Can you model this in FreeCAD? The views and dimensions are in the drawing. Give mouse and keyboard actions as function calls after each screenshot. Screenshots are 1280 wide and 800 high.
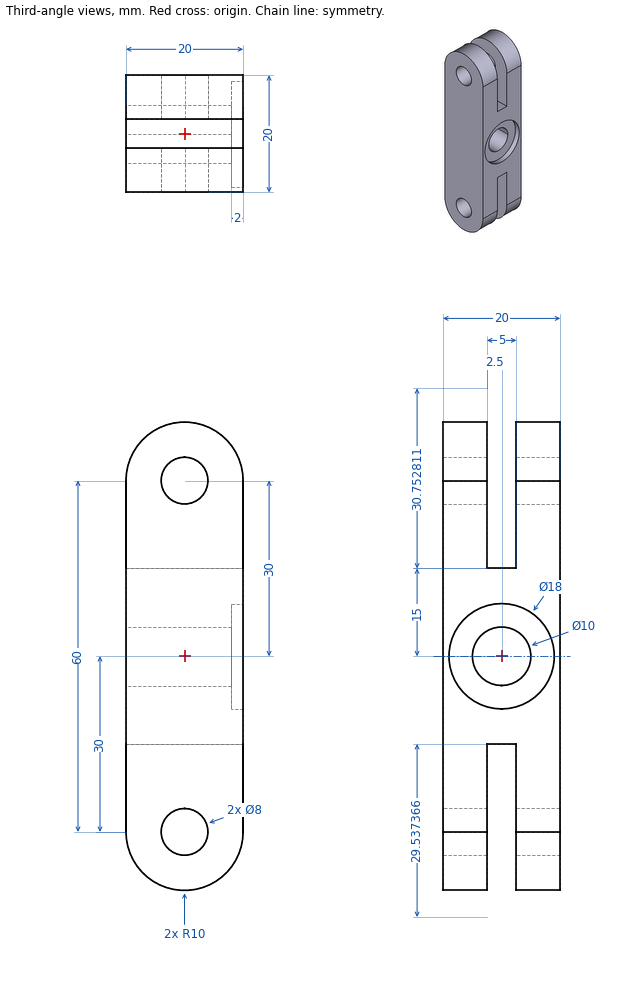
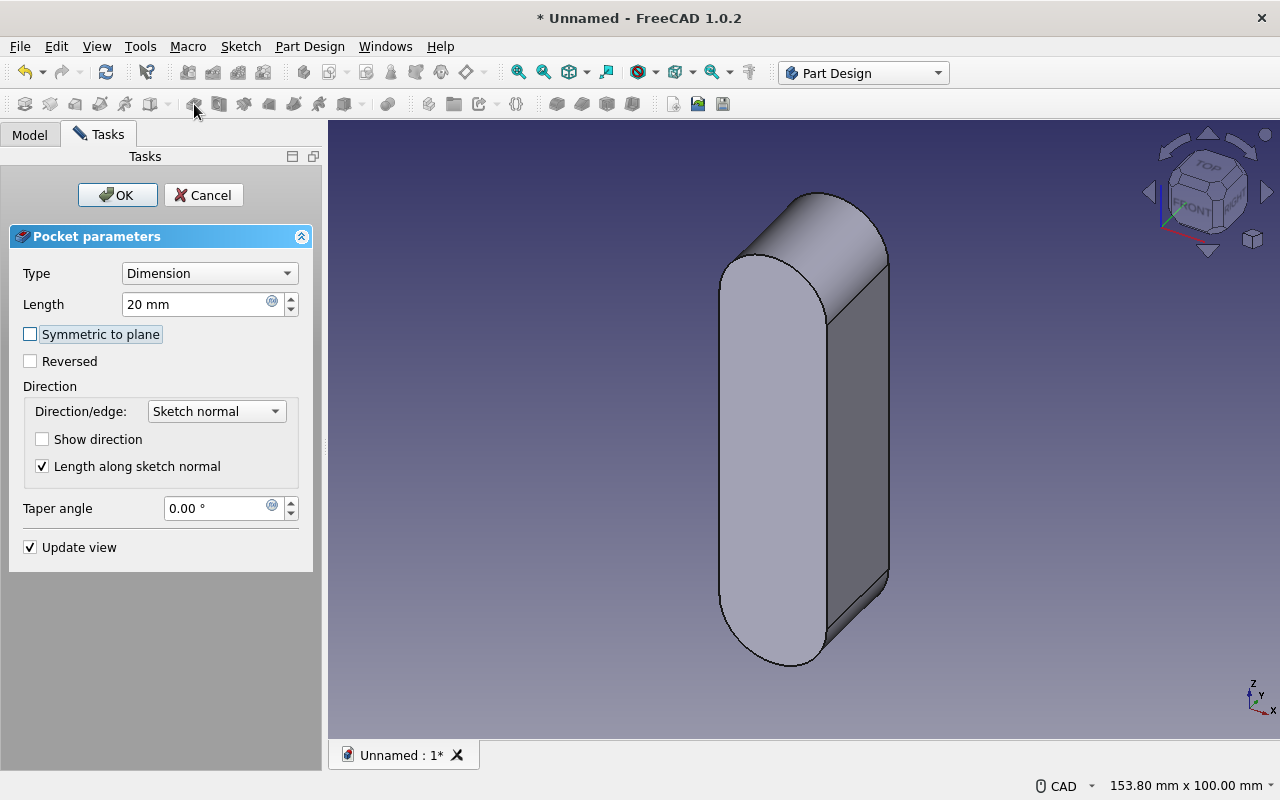
click(31, 334)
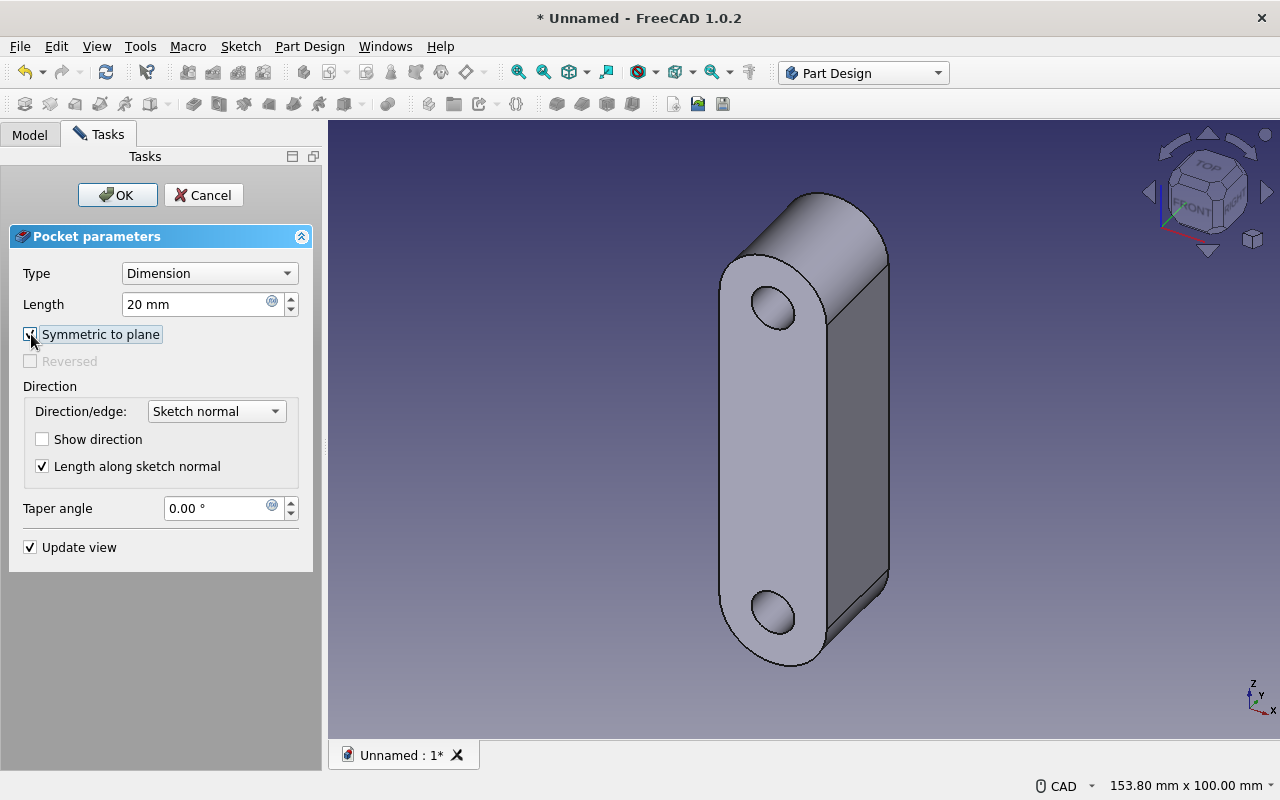
click(118, 195)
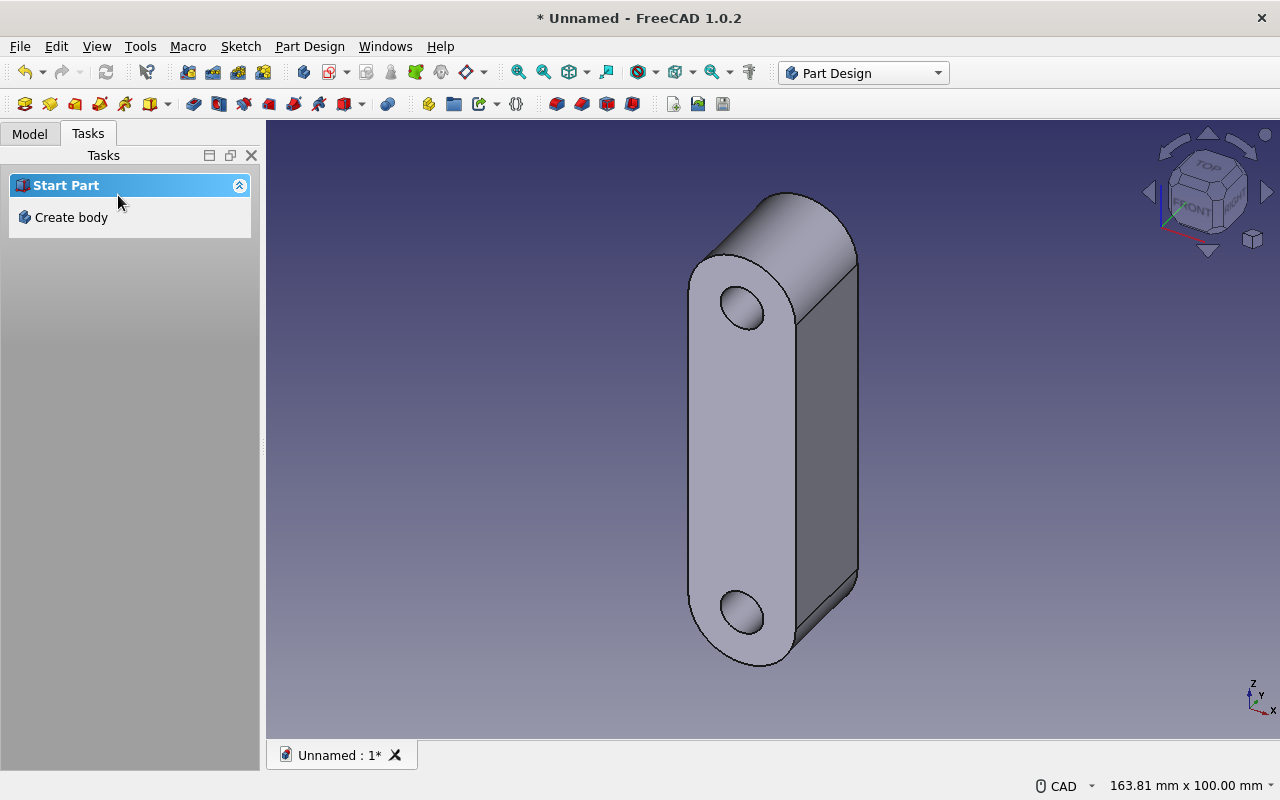
click(328, 72)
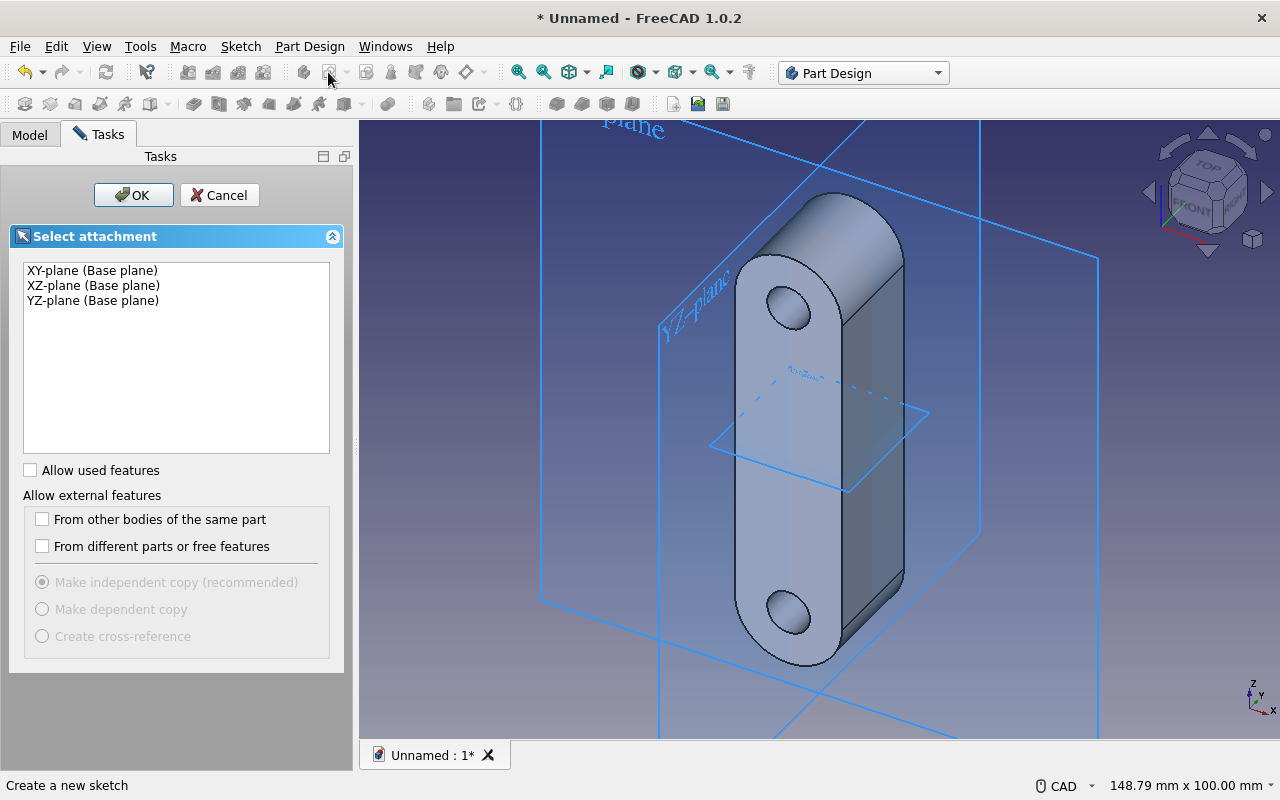
click(84, 300)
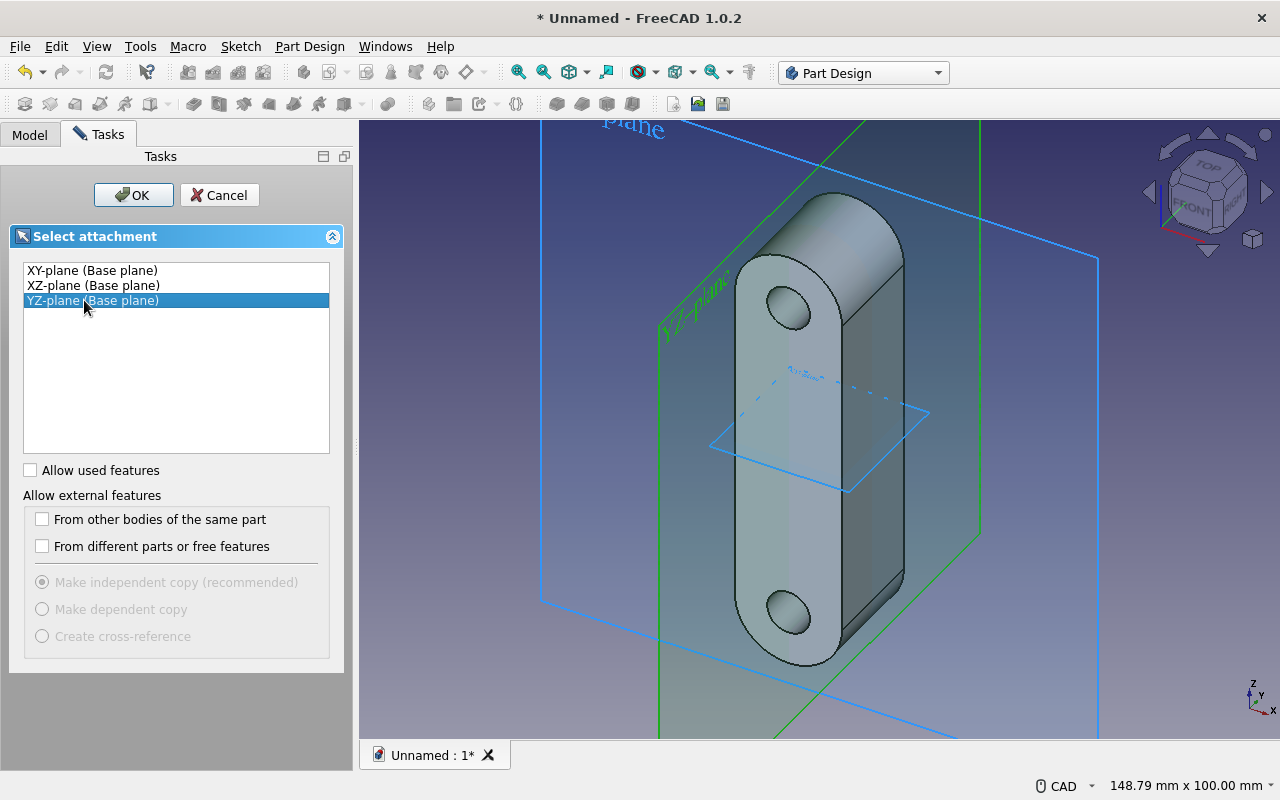
click(134, 195)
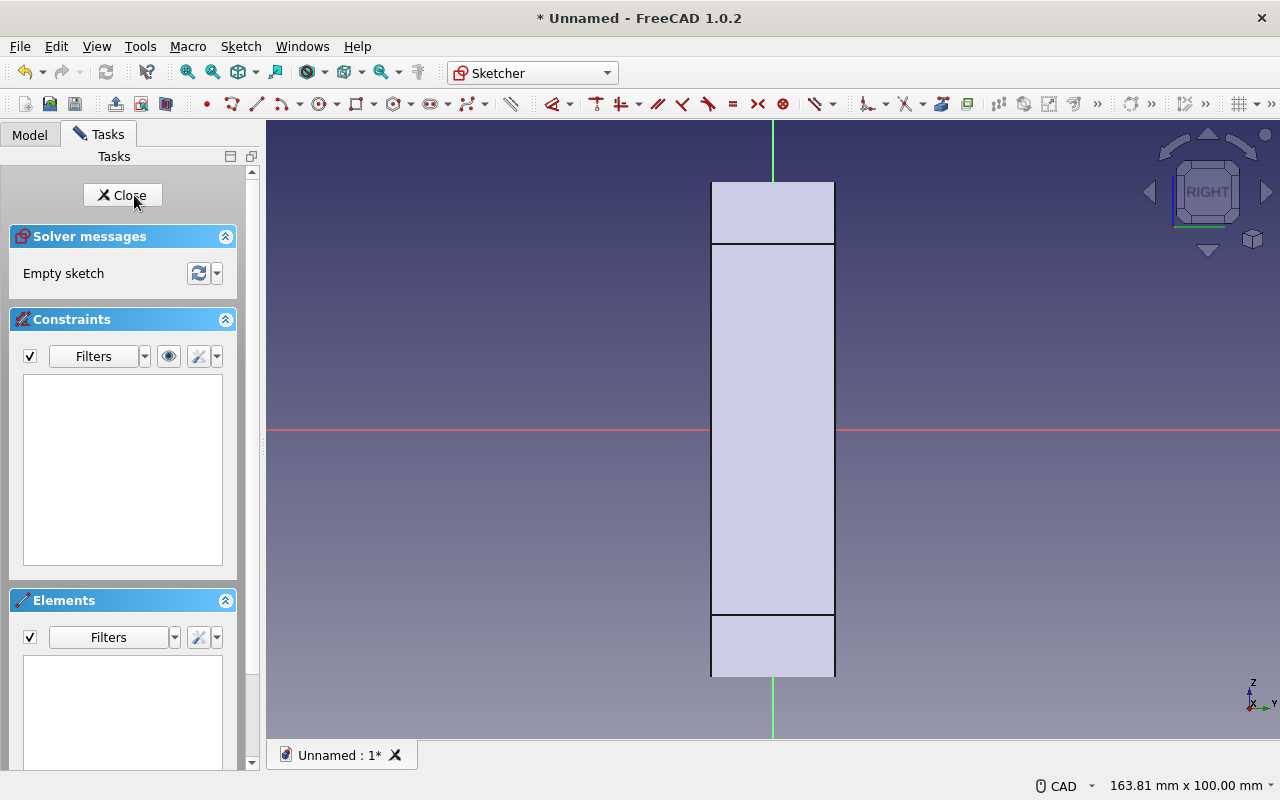
key(q)
key(s)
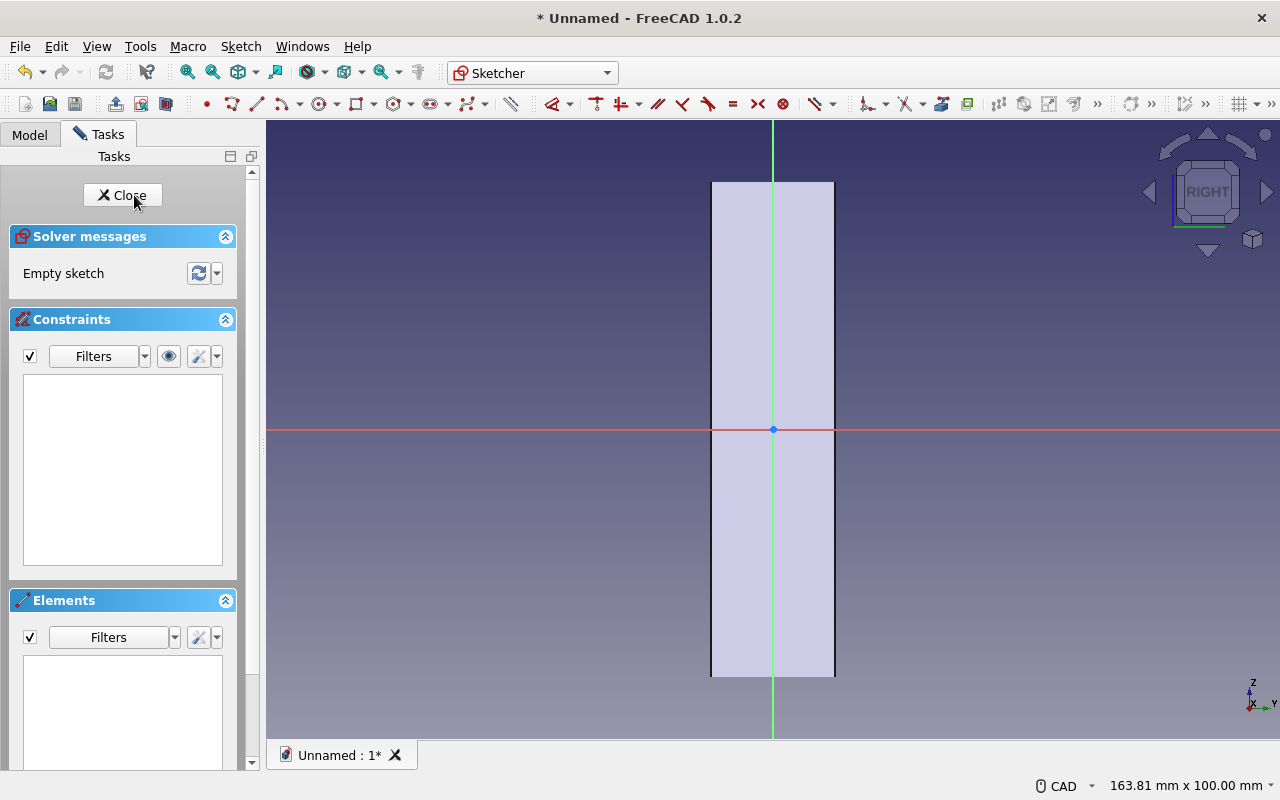
scroll(565, 437, down, 2)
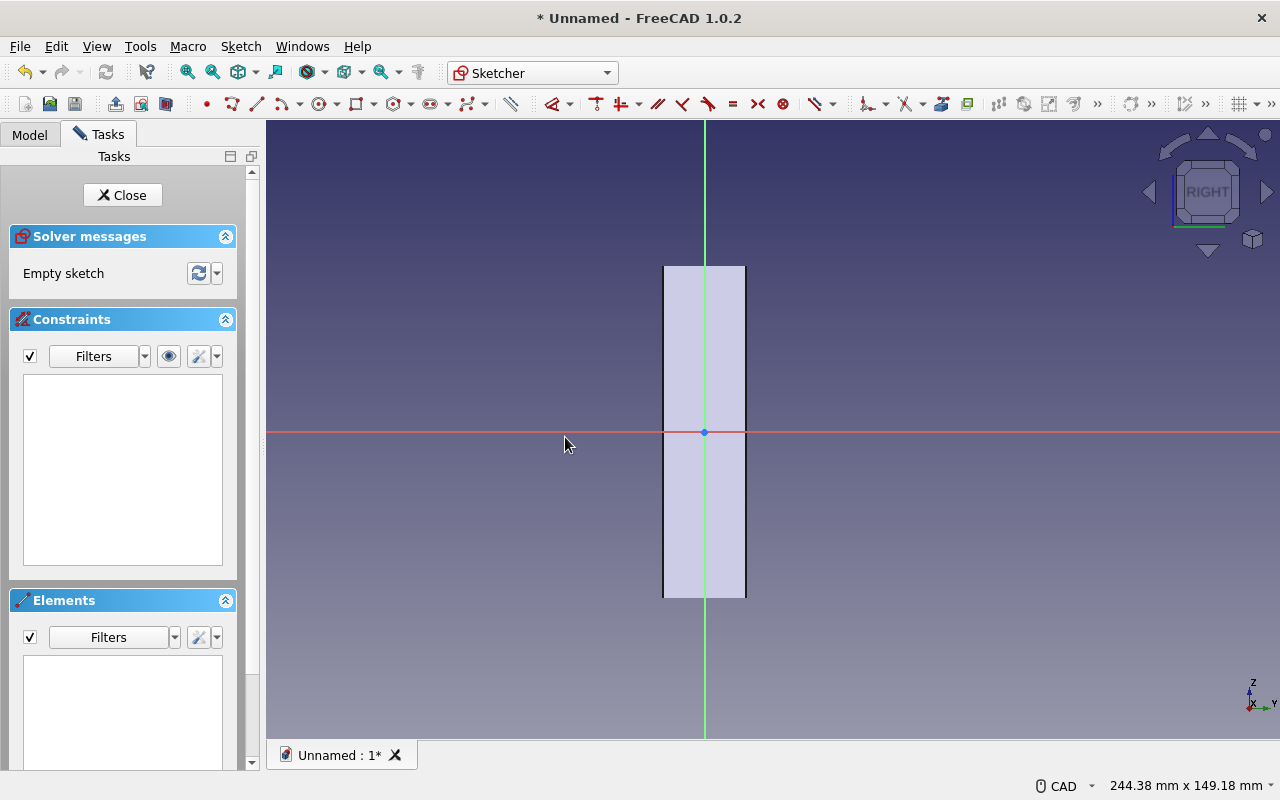
key(g)
key(r)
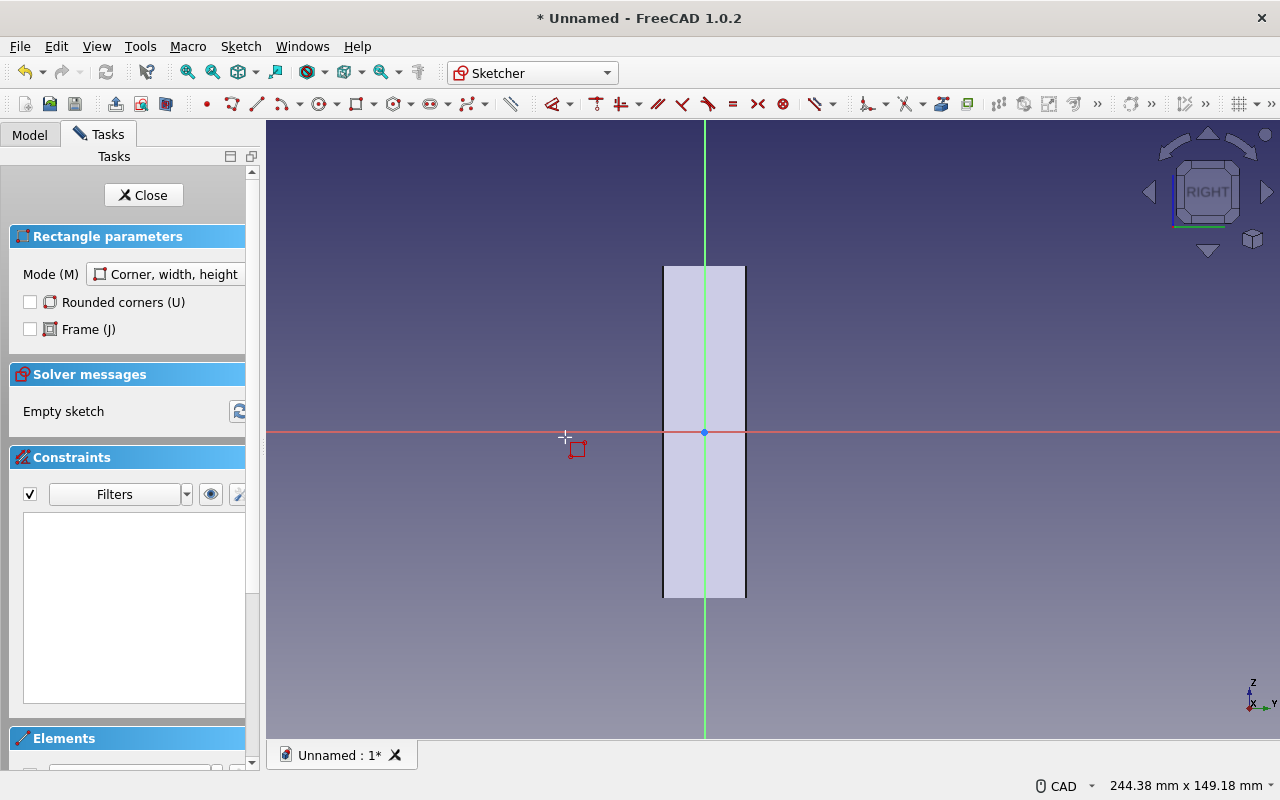
scroll(694, 242, up, 3)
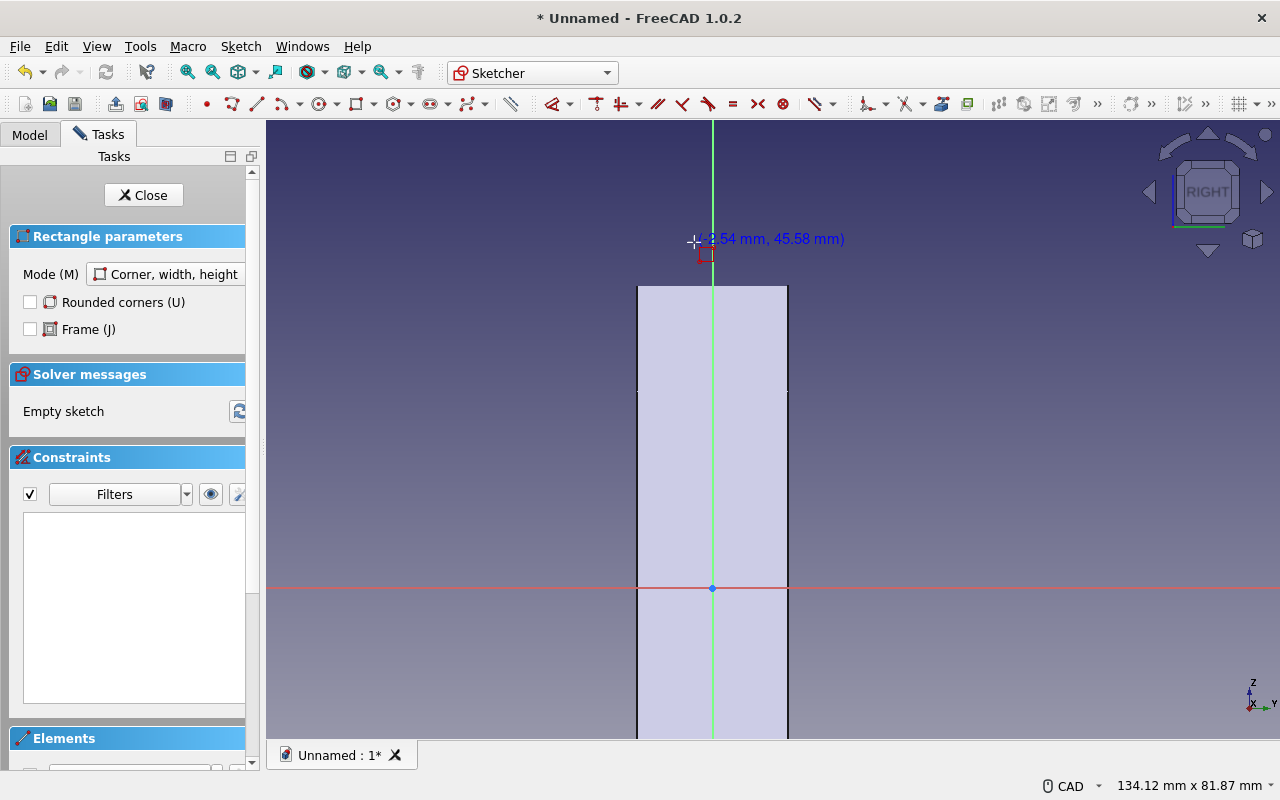
click(694, 242)
click(732, 475)